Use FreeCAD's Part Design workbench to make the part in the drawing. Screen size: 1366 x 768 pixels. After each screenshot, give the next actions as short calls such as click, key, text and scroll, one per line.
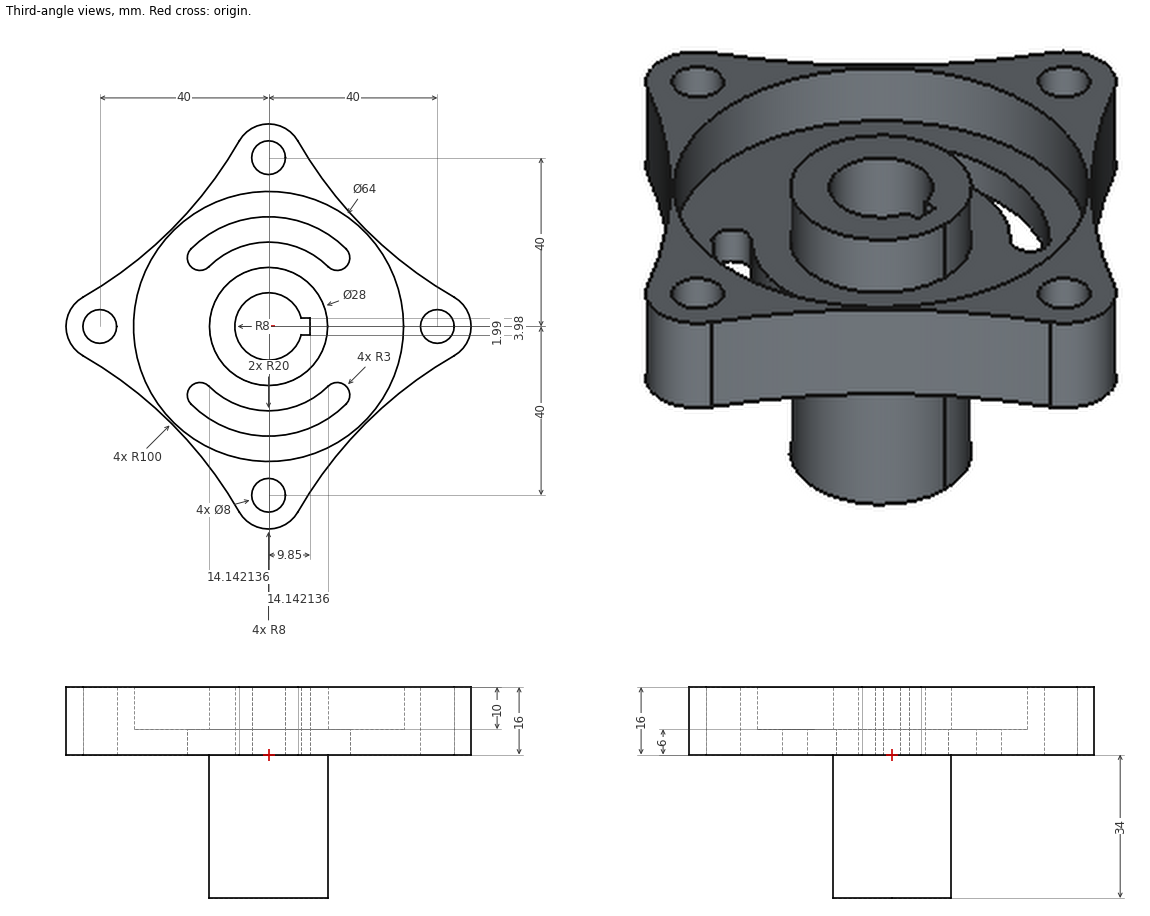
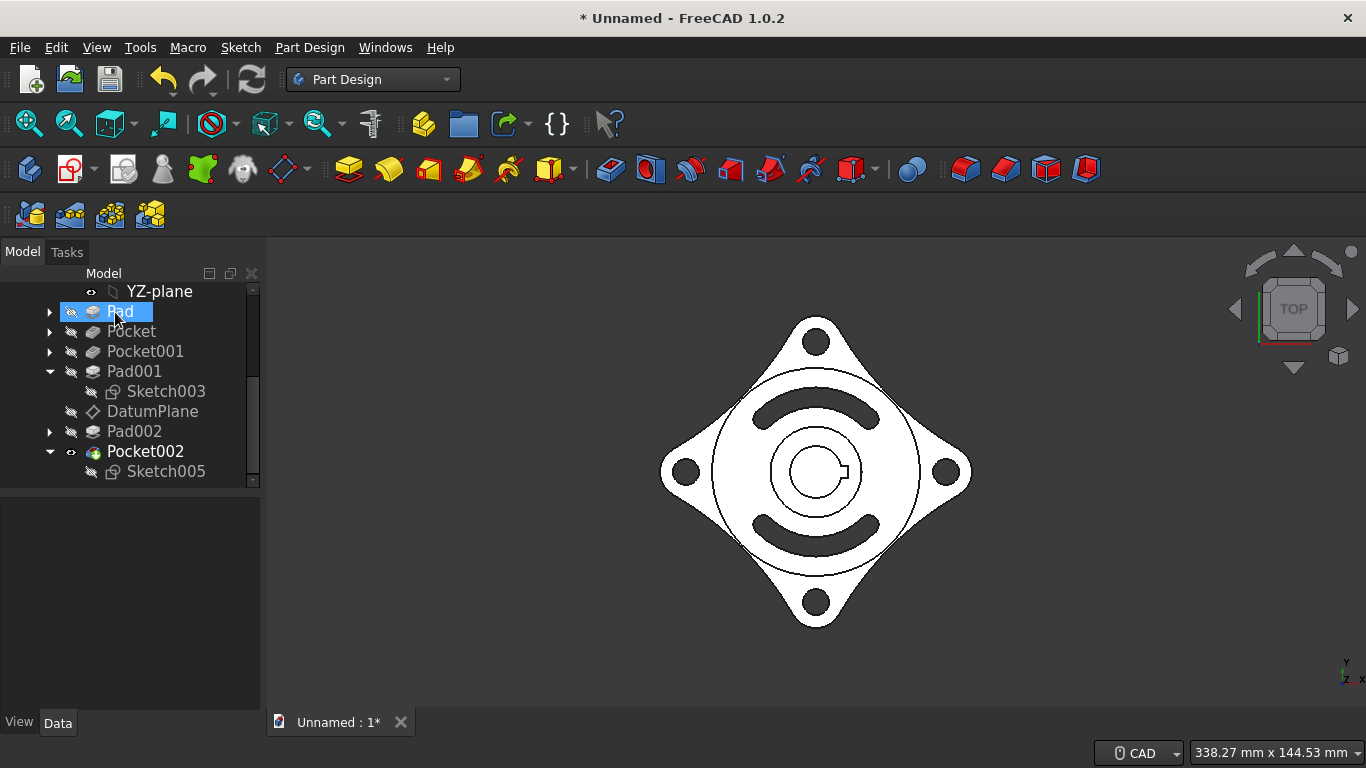
key(0)